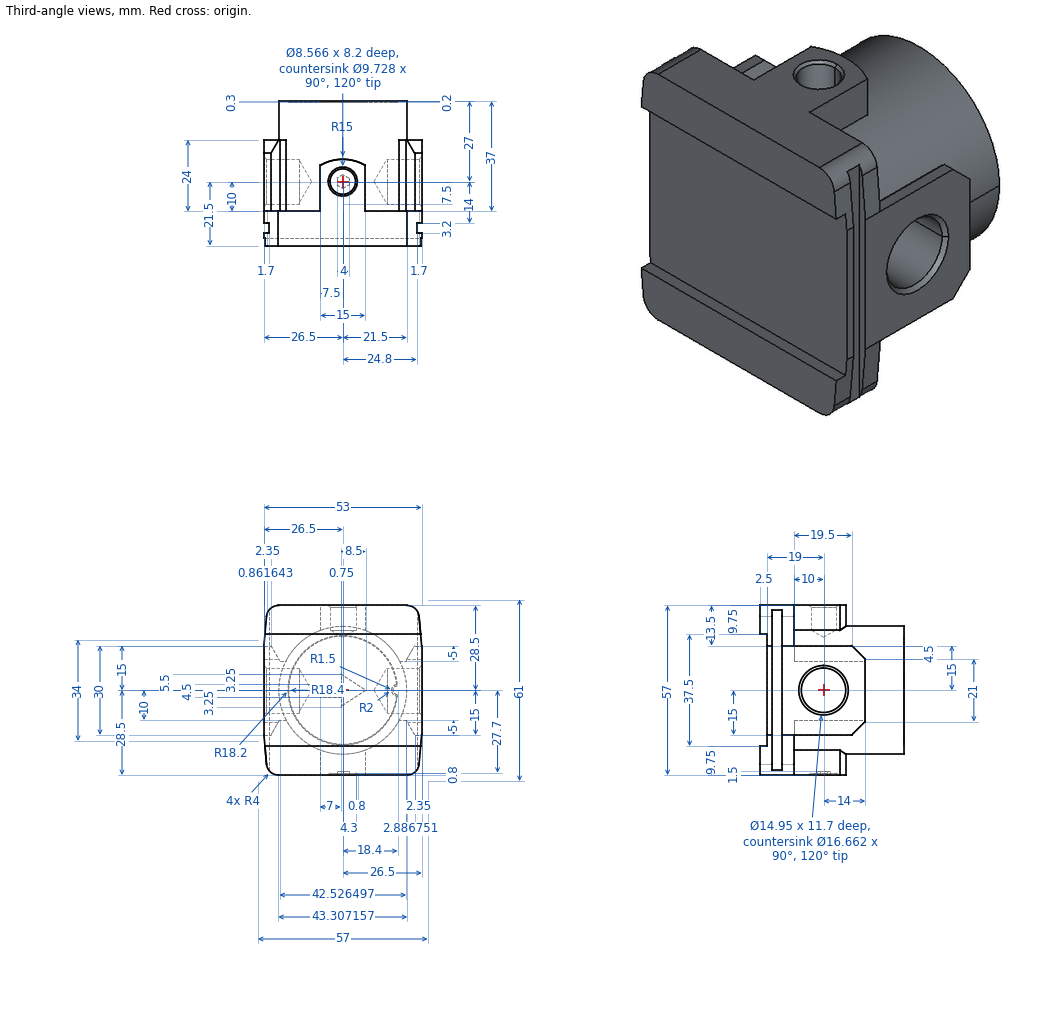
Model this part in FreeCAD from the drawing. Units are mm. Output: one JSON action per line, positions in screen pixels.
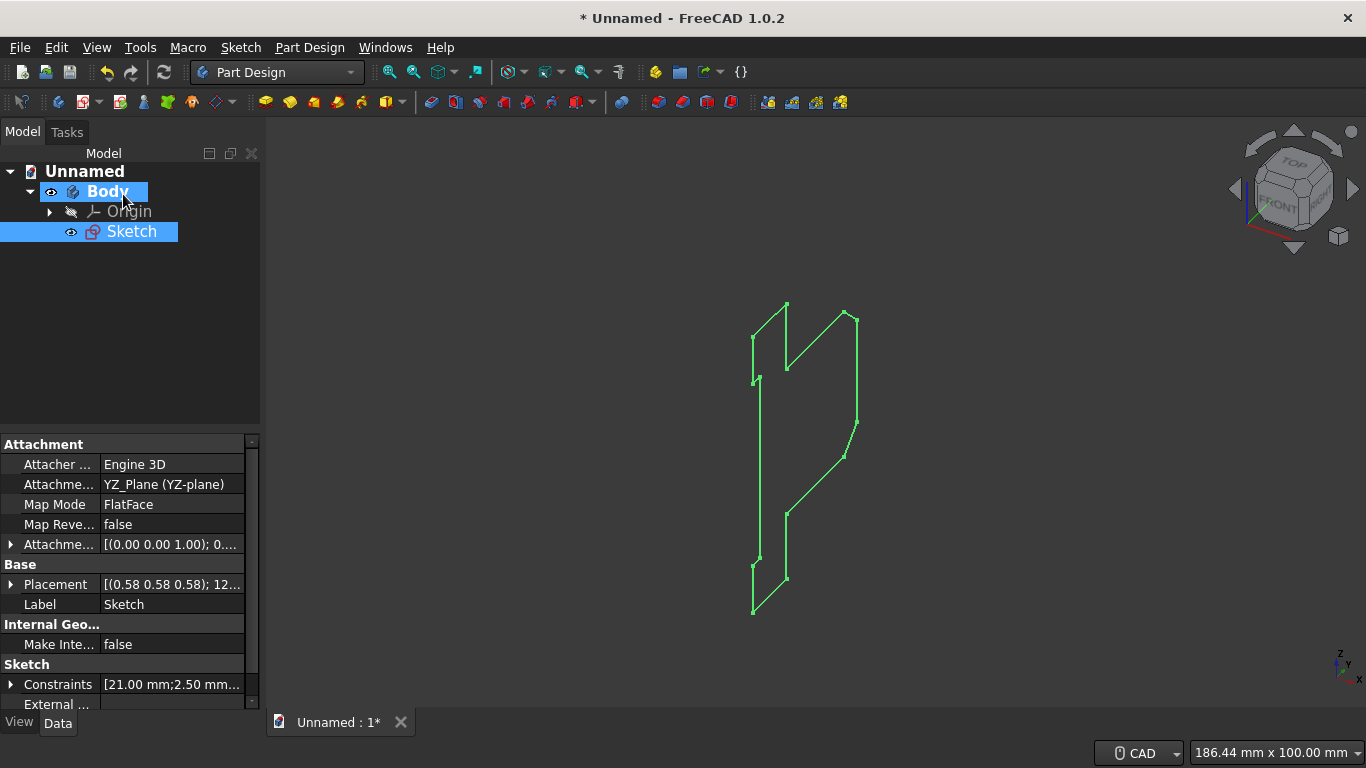
{"action": "left_click", "coordinate": [266, 102]}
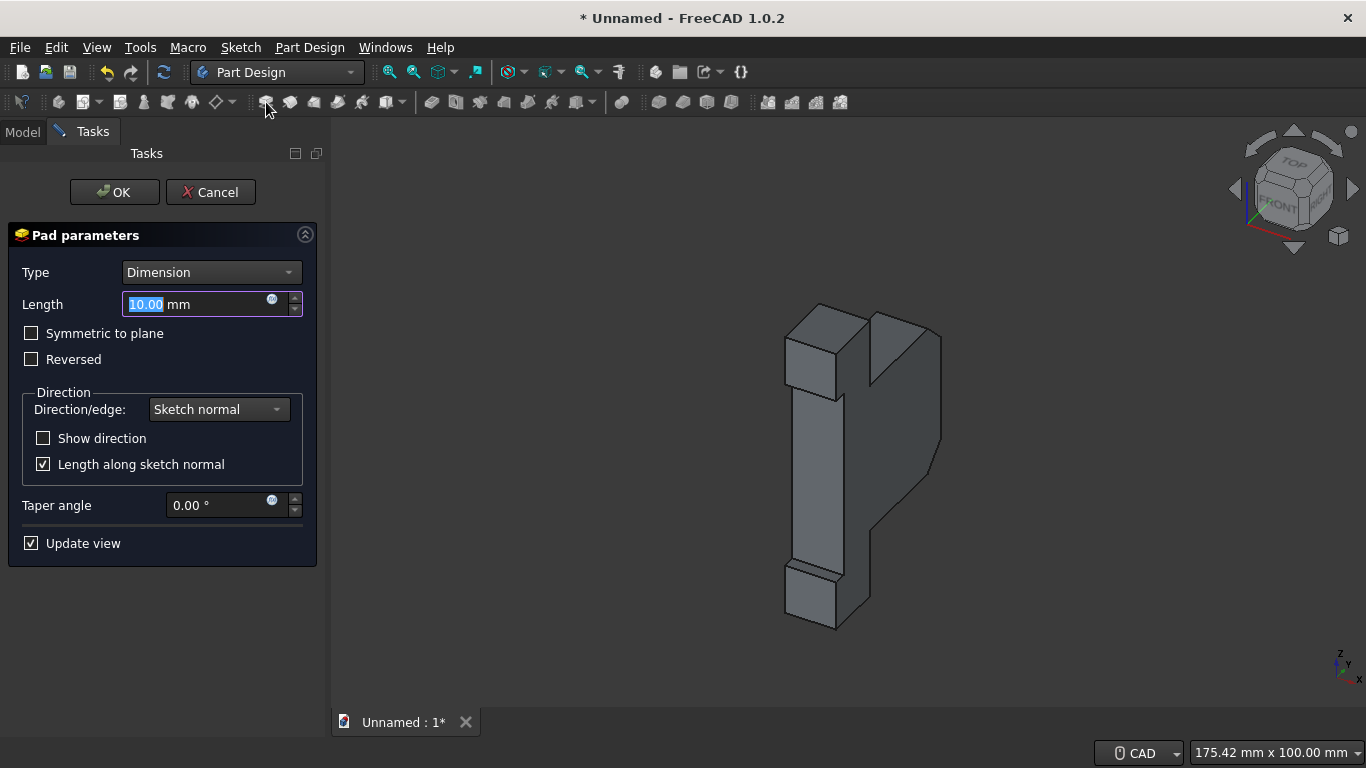
{"action": "type", "text": "53"}
{"action": "key", "text": "Tab"}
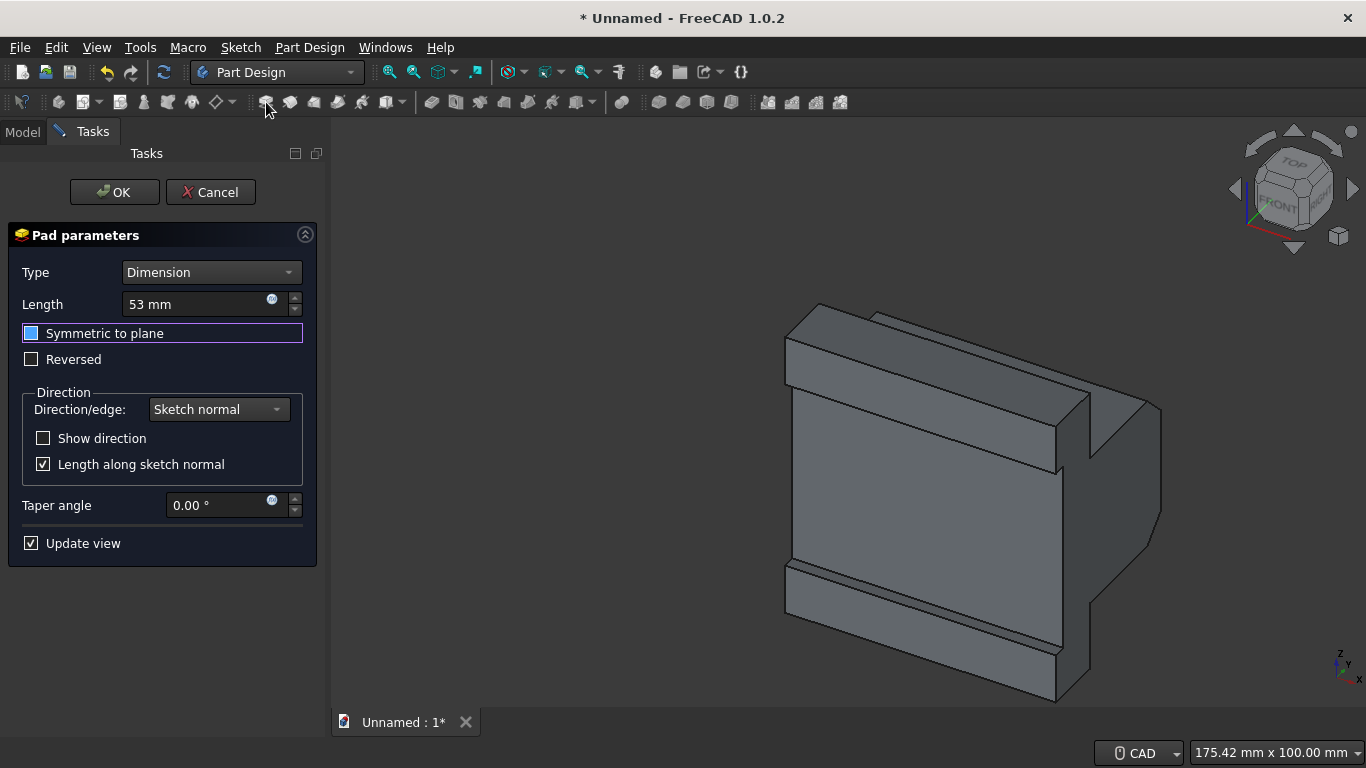
{"action": "left_click", "coordinate": [30, 333]}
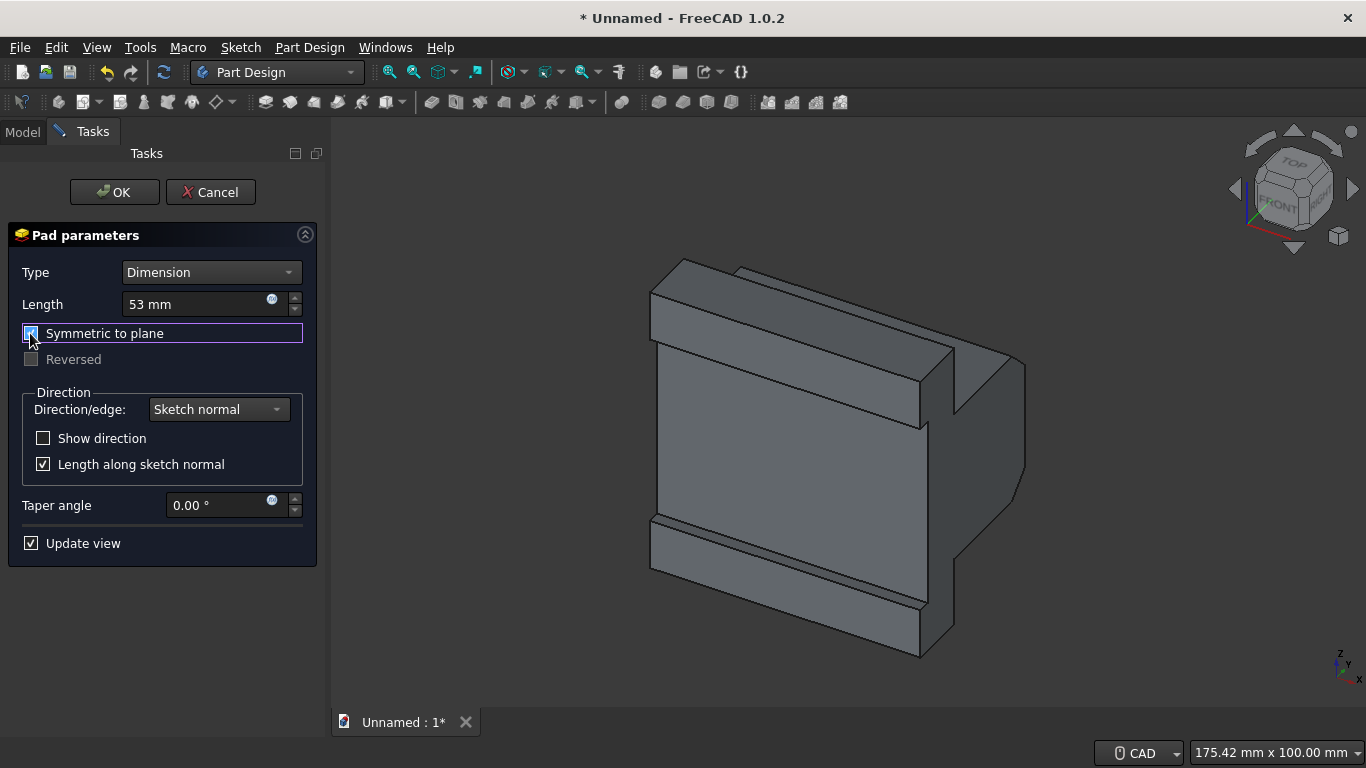
{"action": "left_click", "coordinate": [115, 192]}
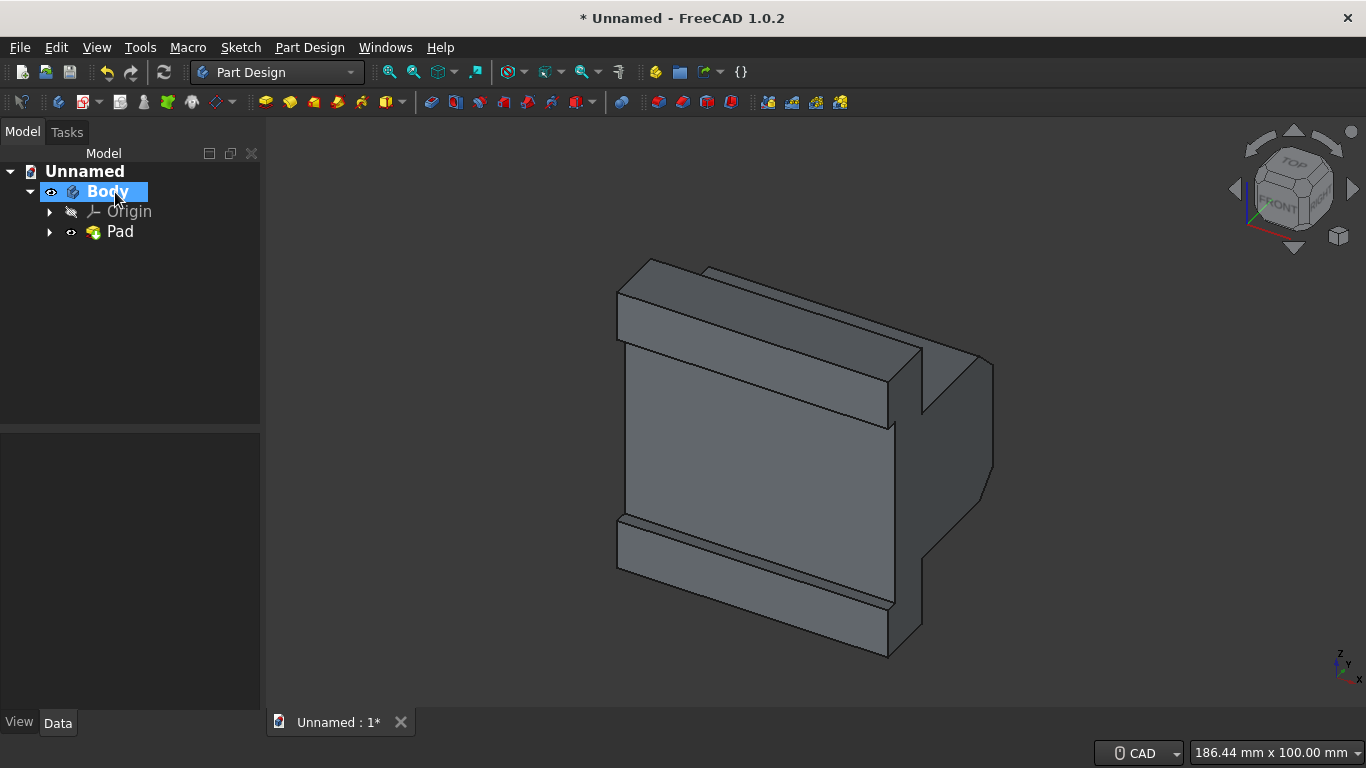
{"action": "left_click", "coordinate": [84, 102]}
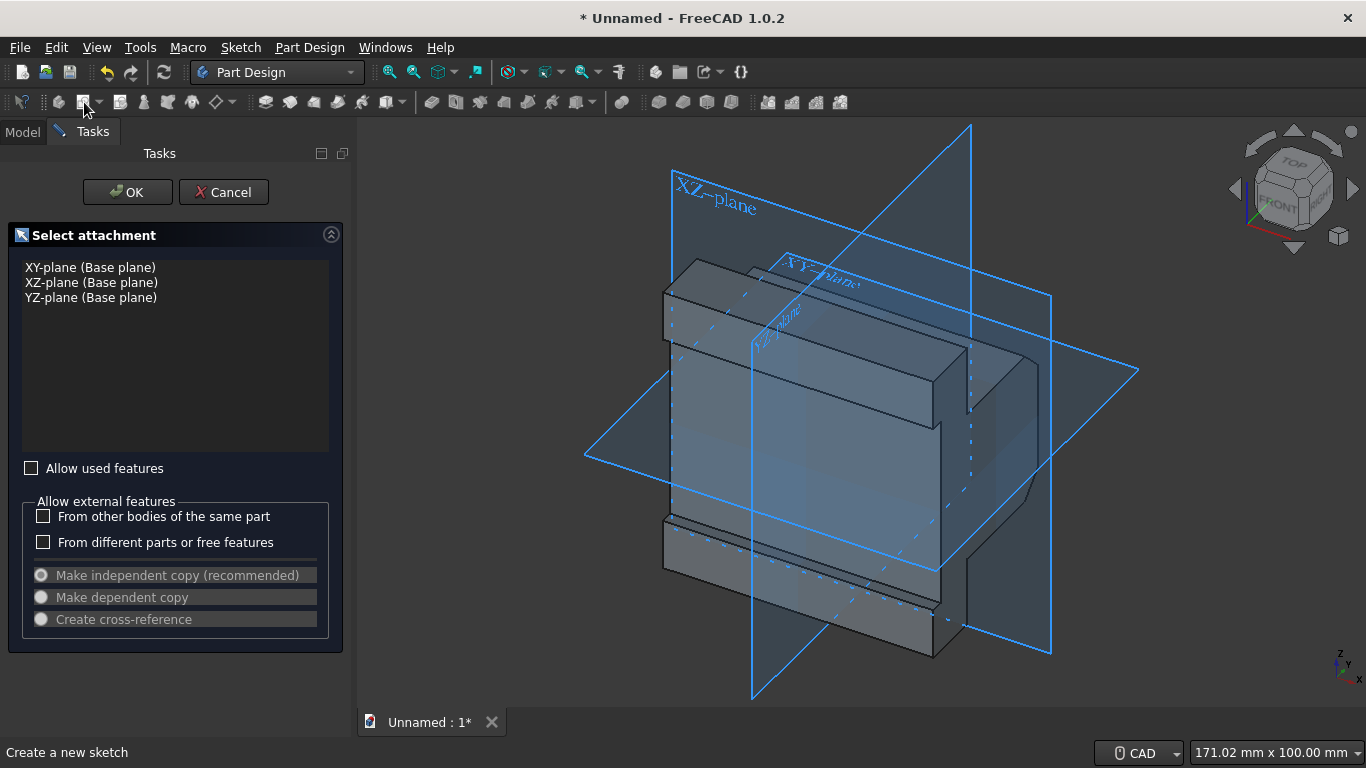
{"action": "left_click", "coordinate": [82, 282]}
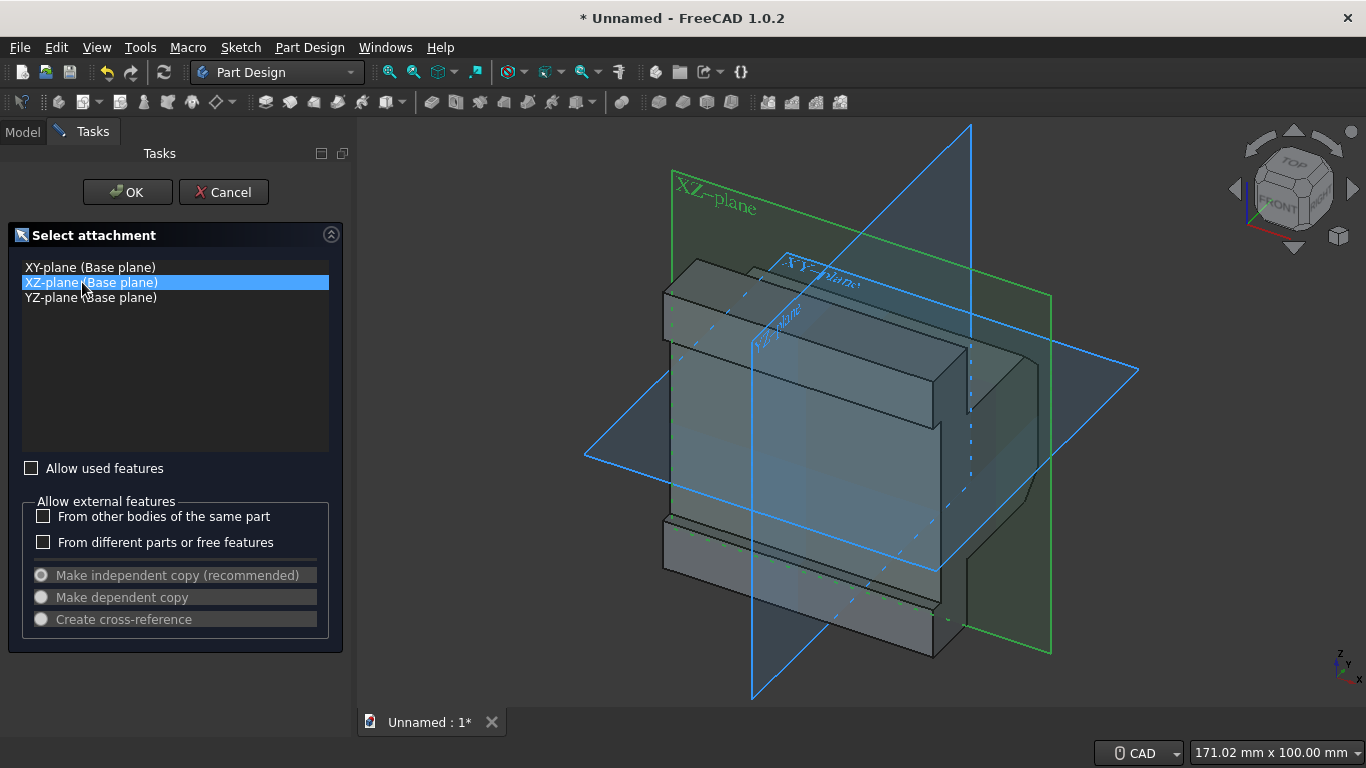
{"action": "left_click", "coordinate": [128, 192]}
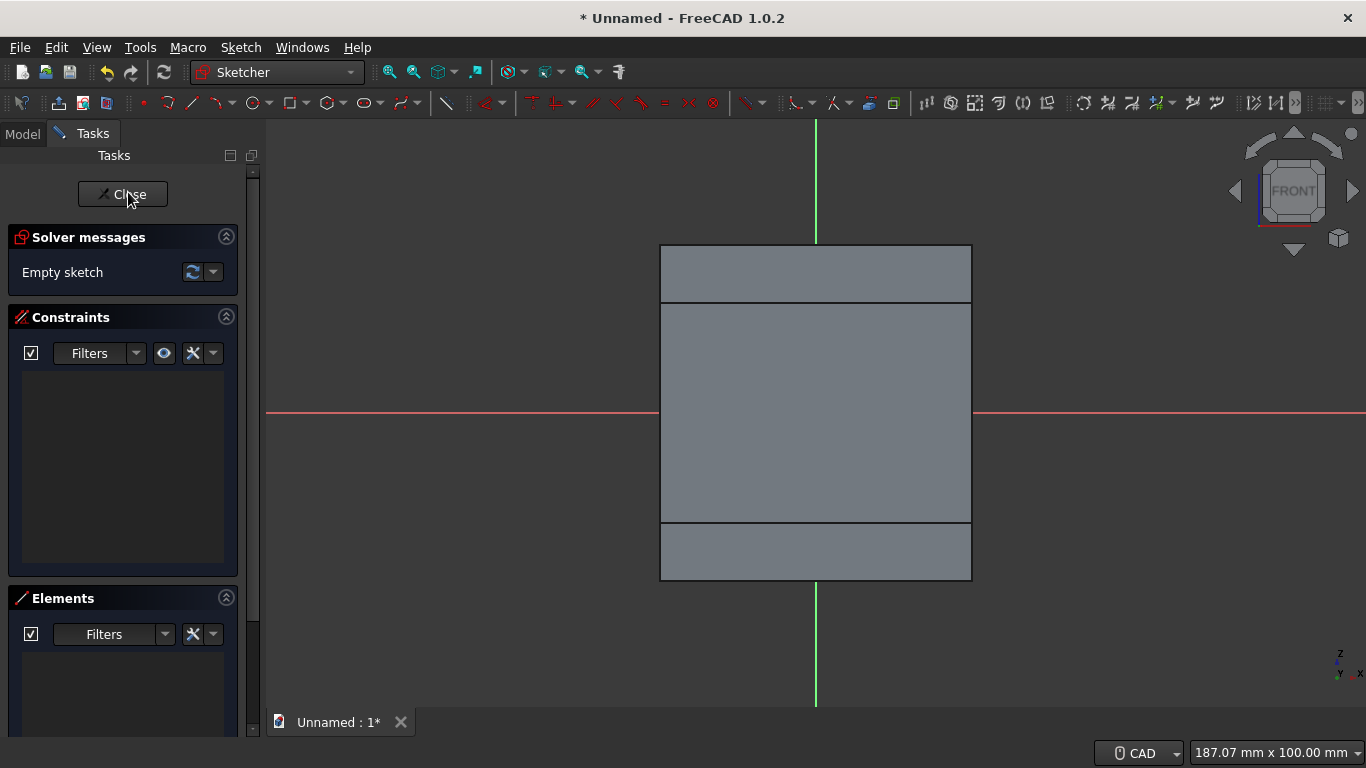
{"action": "left_click", "coordinate": [108, 104]}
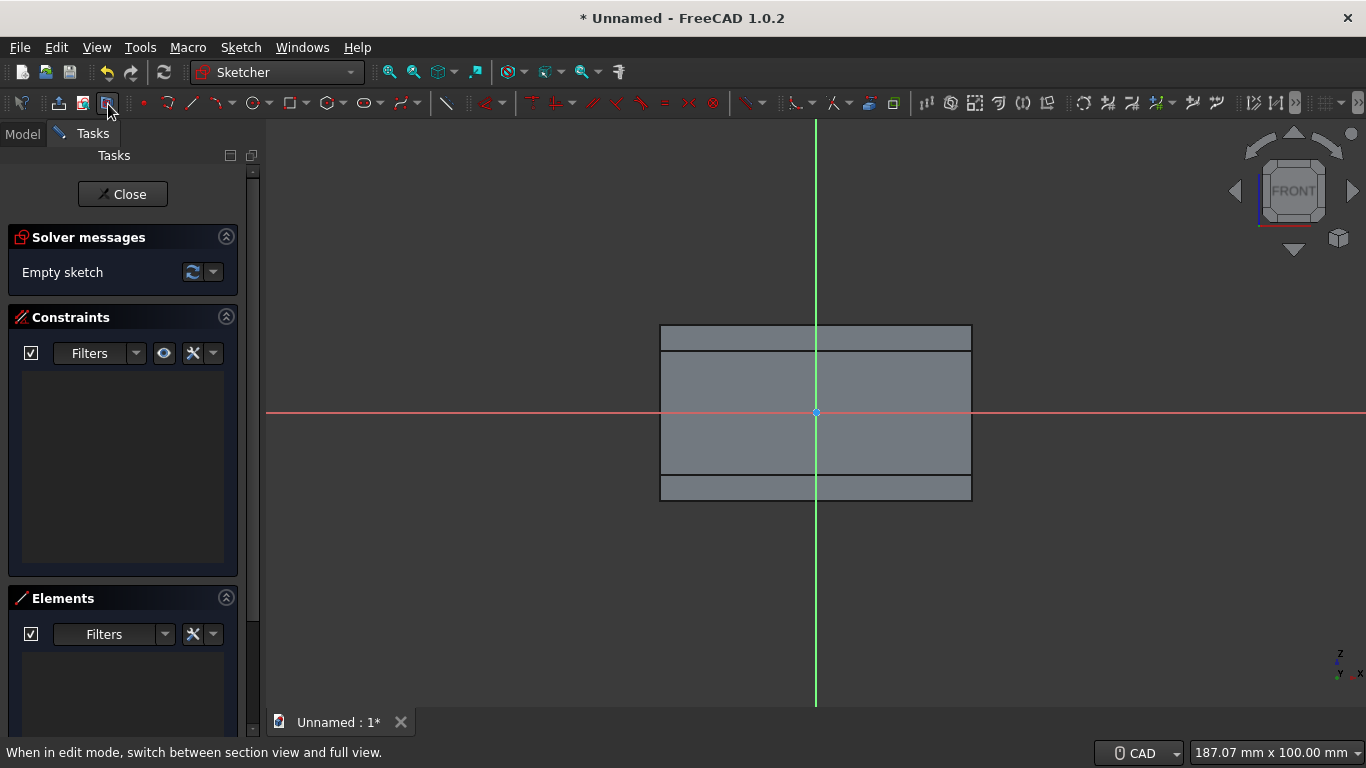
{"action": "left_click", "coordinate": [308, 104]}